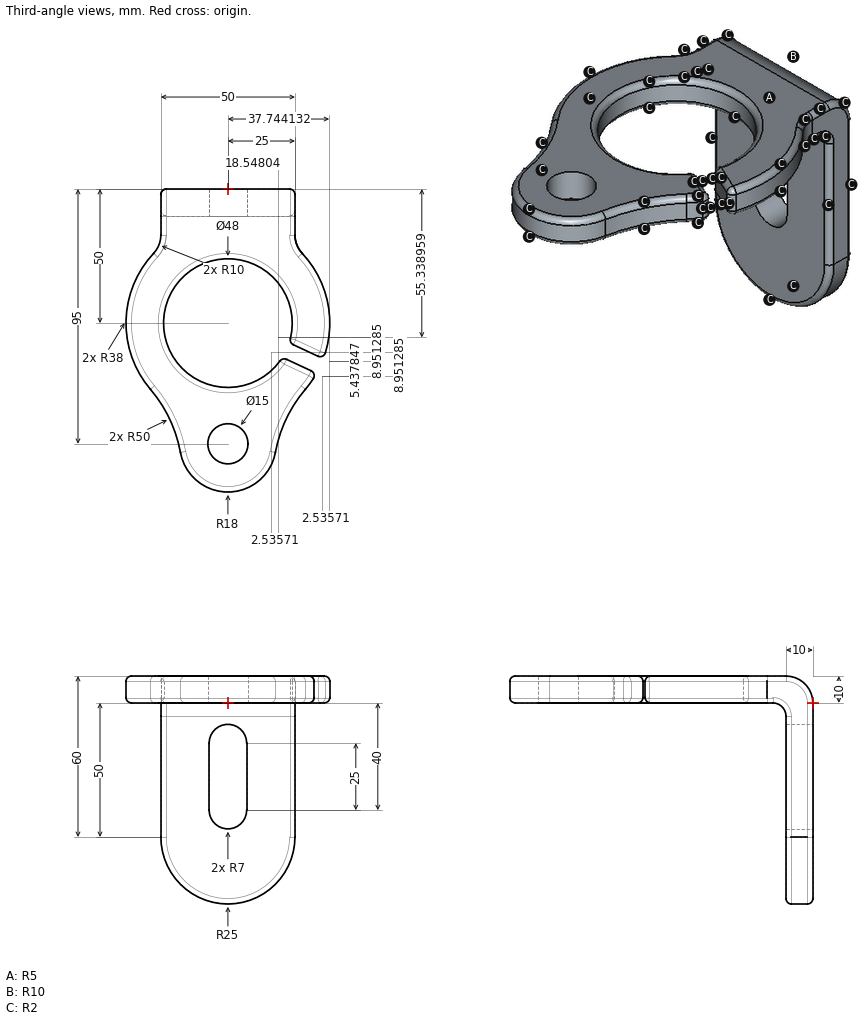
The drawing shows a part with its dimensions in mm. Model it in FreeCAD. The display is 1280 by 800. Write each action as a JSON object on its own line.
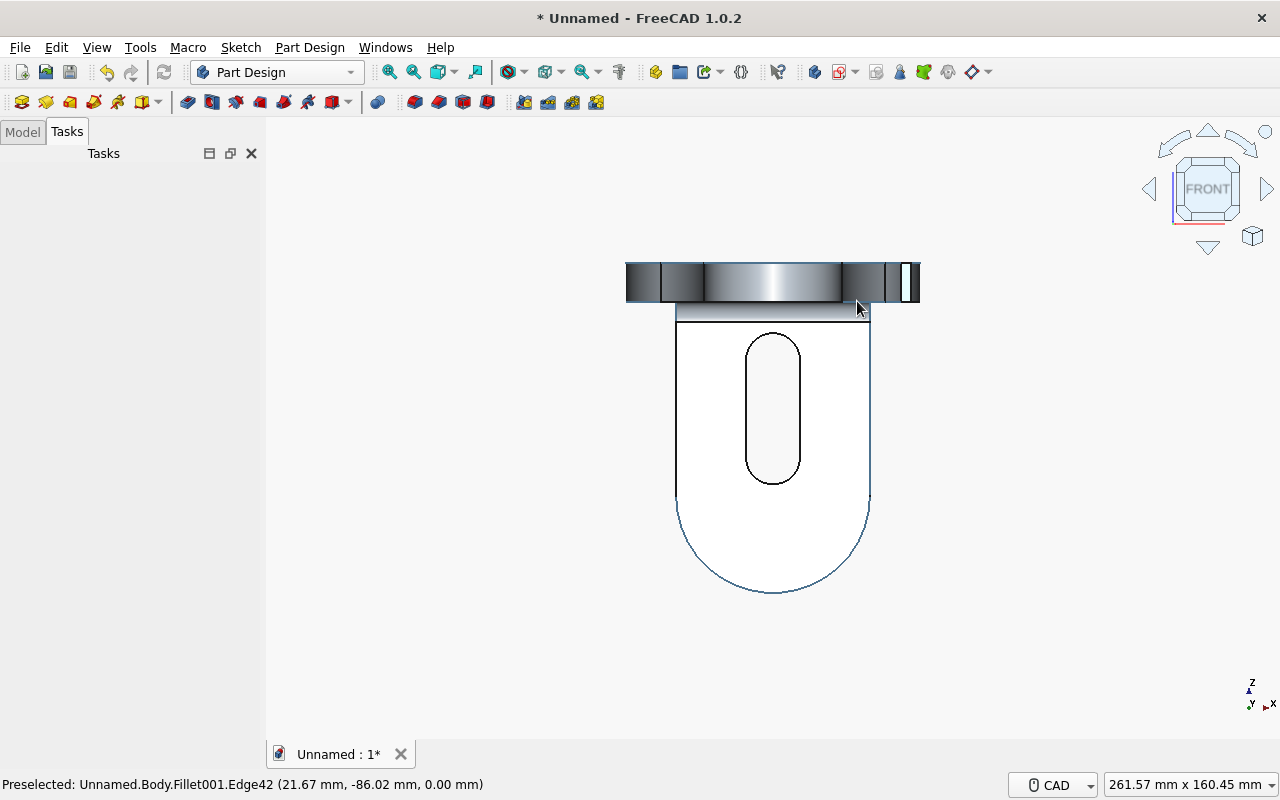
{"action": "left_click", "coordinate": [773, 301], "text": "ctrl"}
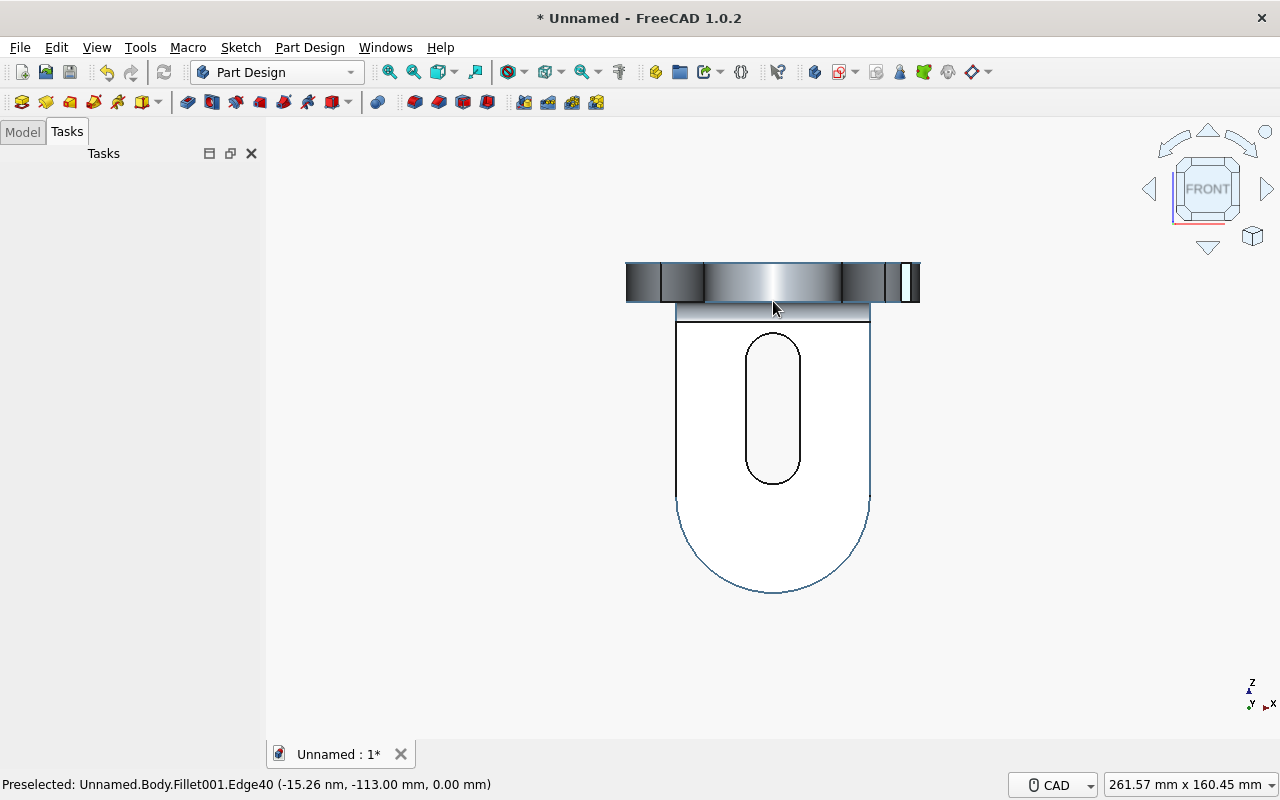
{"action": "left_click", "coordinate": [689, 301], "text": "ctrl"}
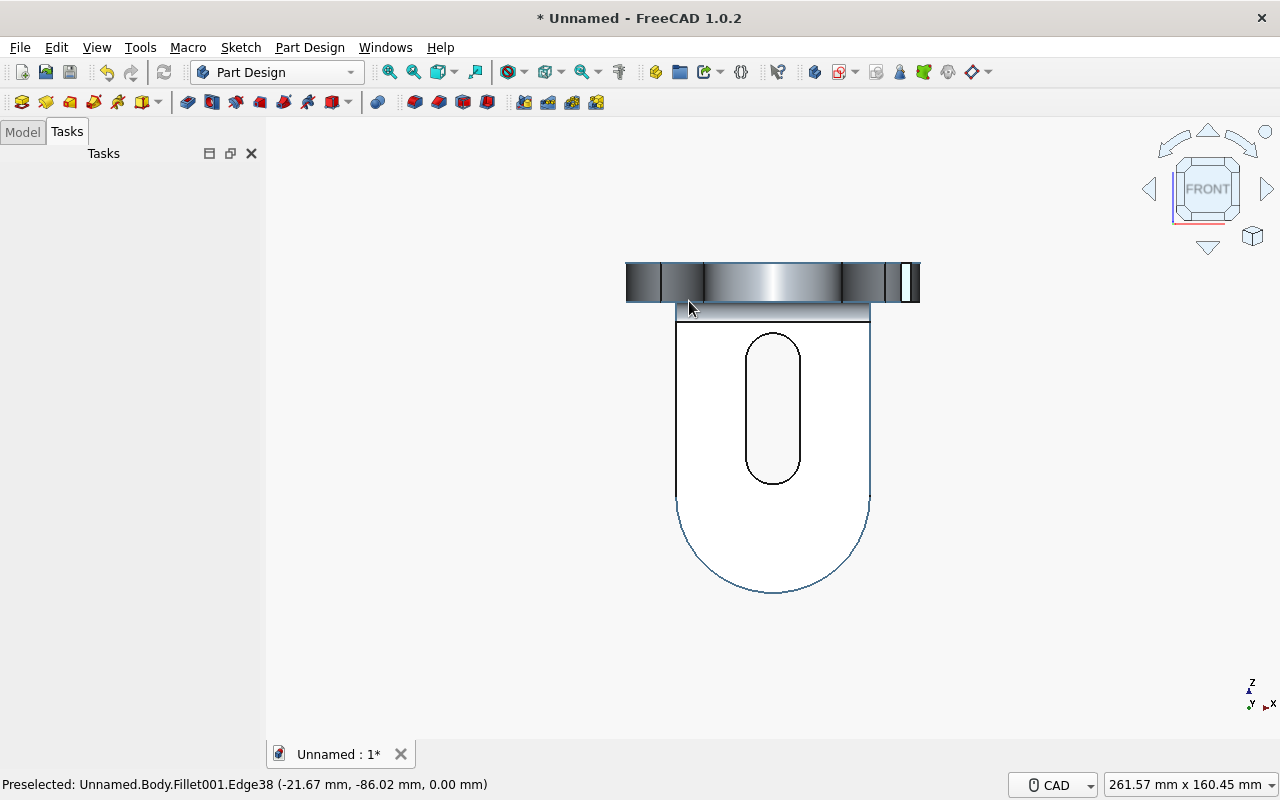
{"action": "left_click", "coordinate": [676, 408], "text": "ctrl"}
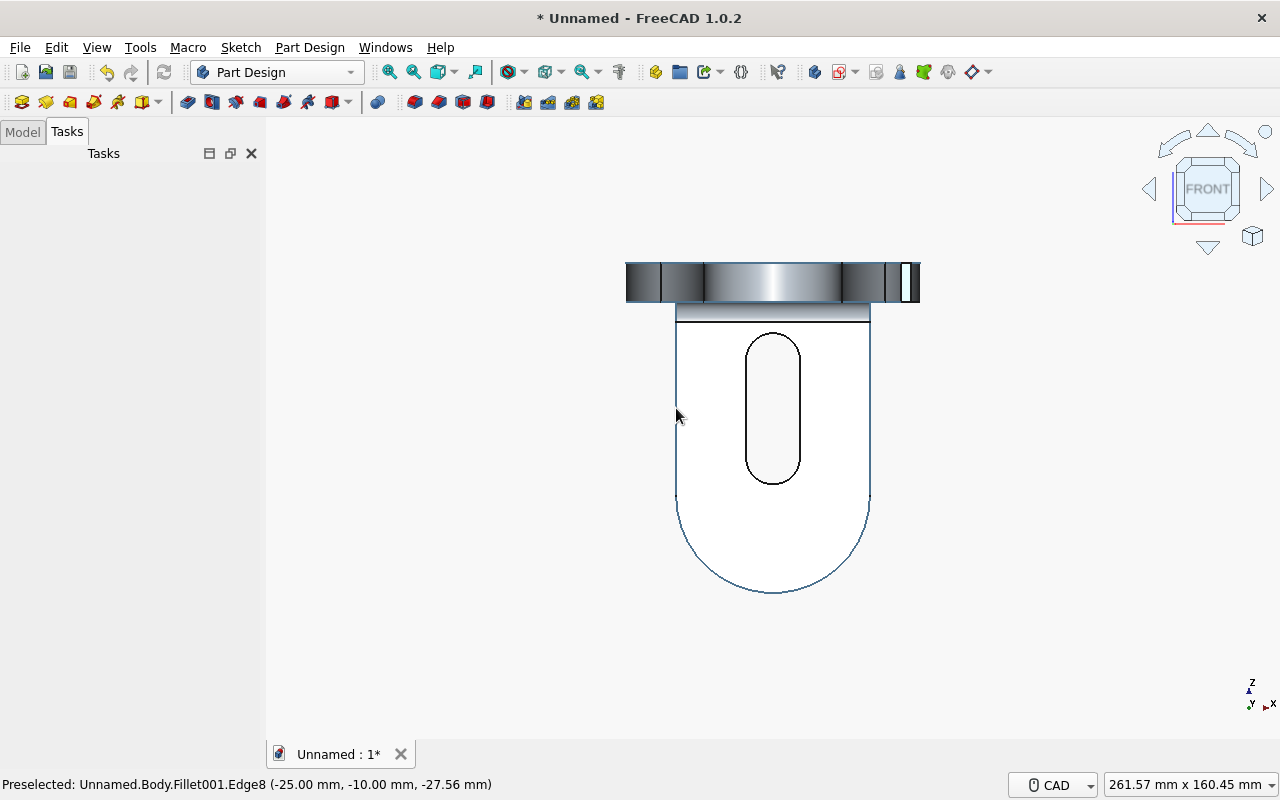
{"action": "left_click", "coordinate": [919, 301], "text": "ctrl"}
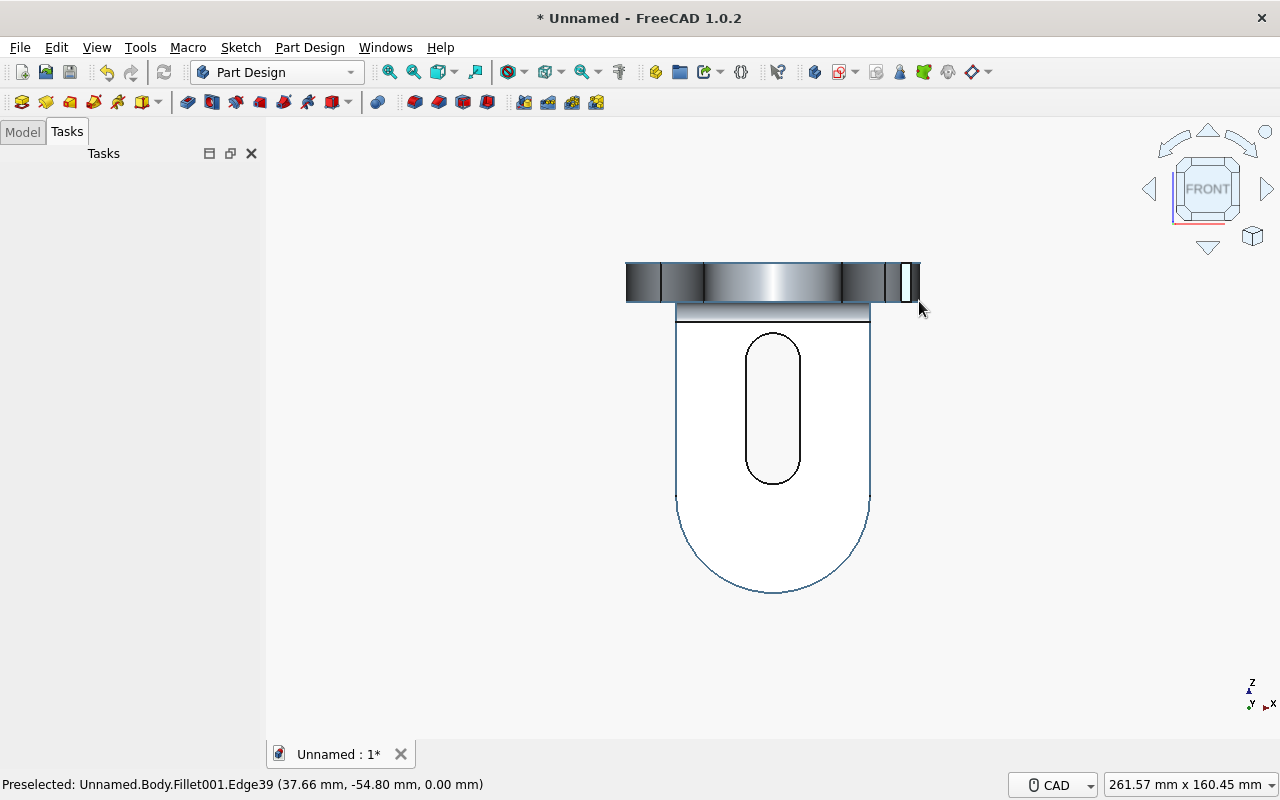
{"action": "key", "text": "3"}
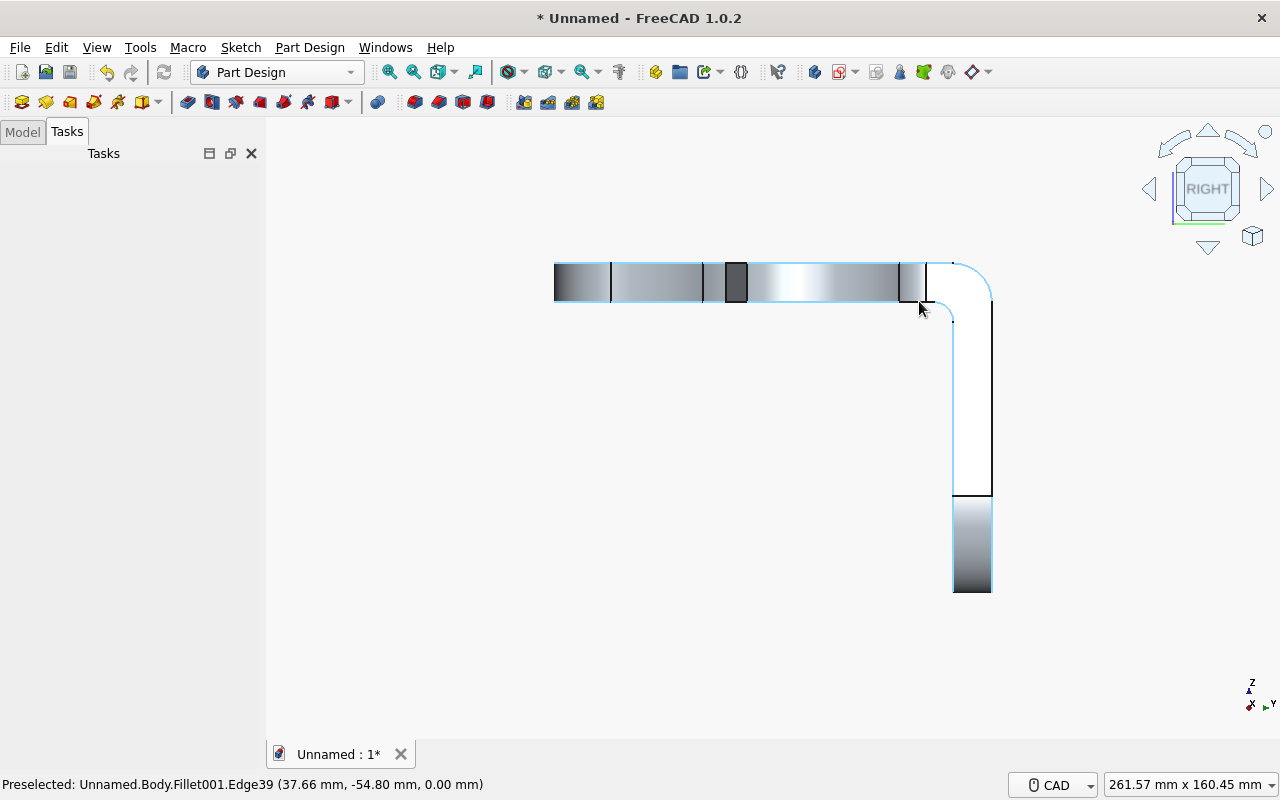
{"action": "left_click", "coordinate": [734, 282], "text": "ctrl"}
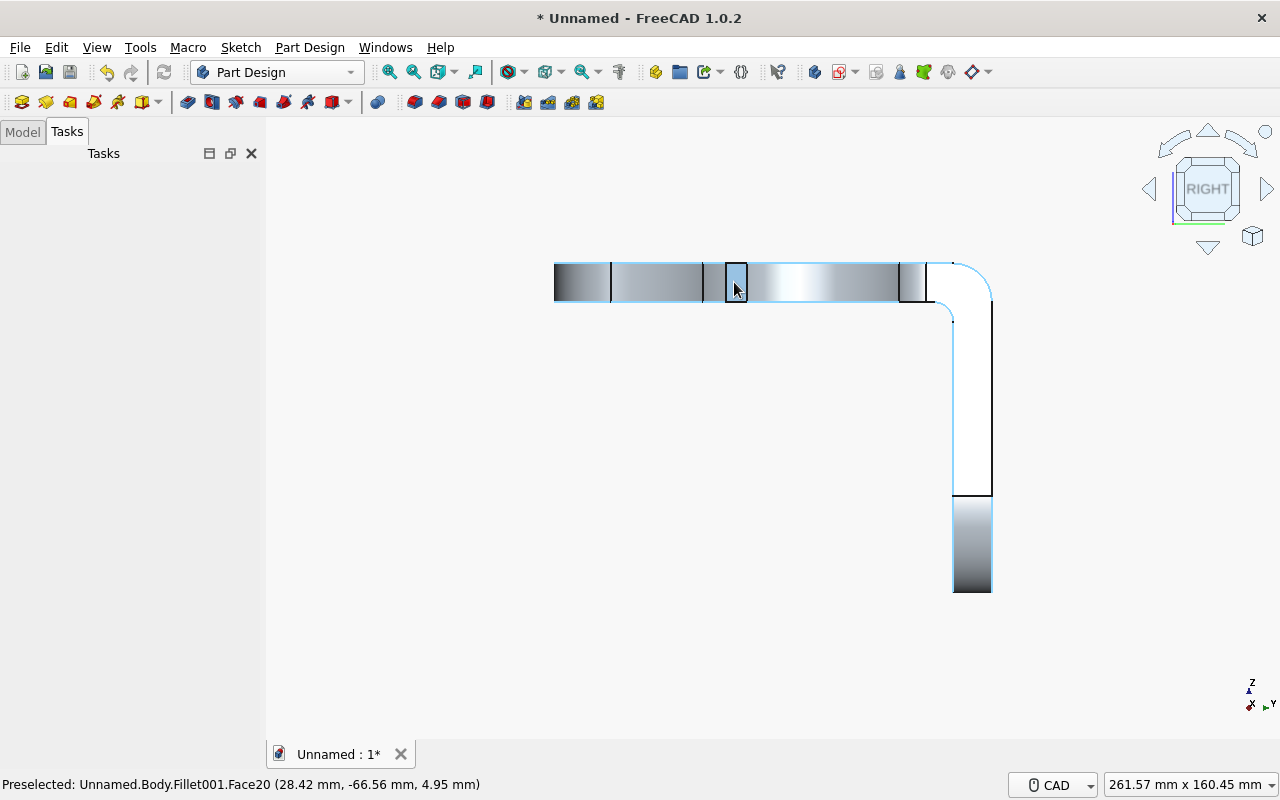
{"action": "left_click", "coordinate": [992, 398], "text": "ctrl"}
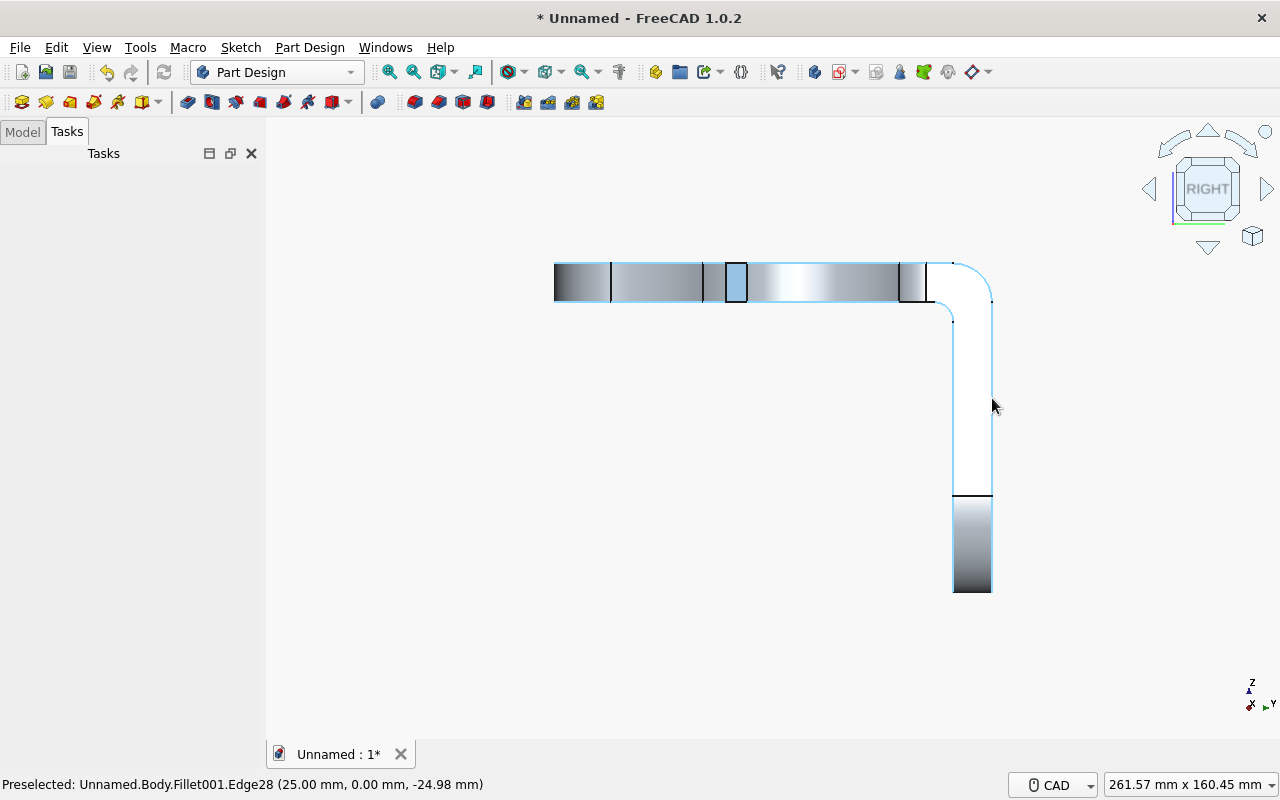
{"action": "left_click", "coordinate": [911, 301], "text": "ctrl"}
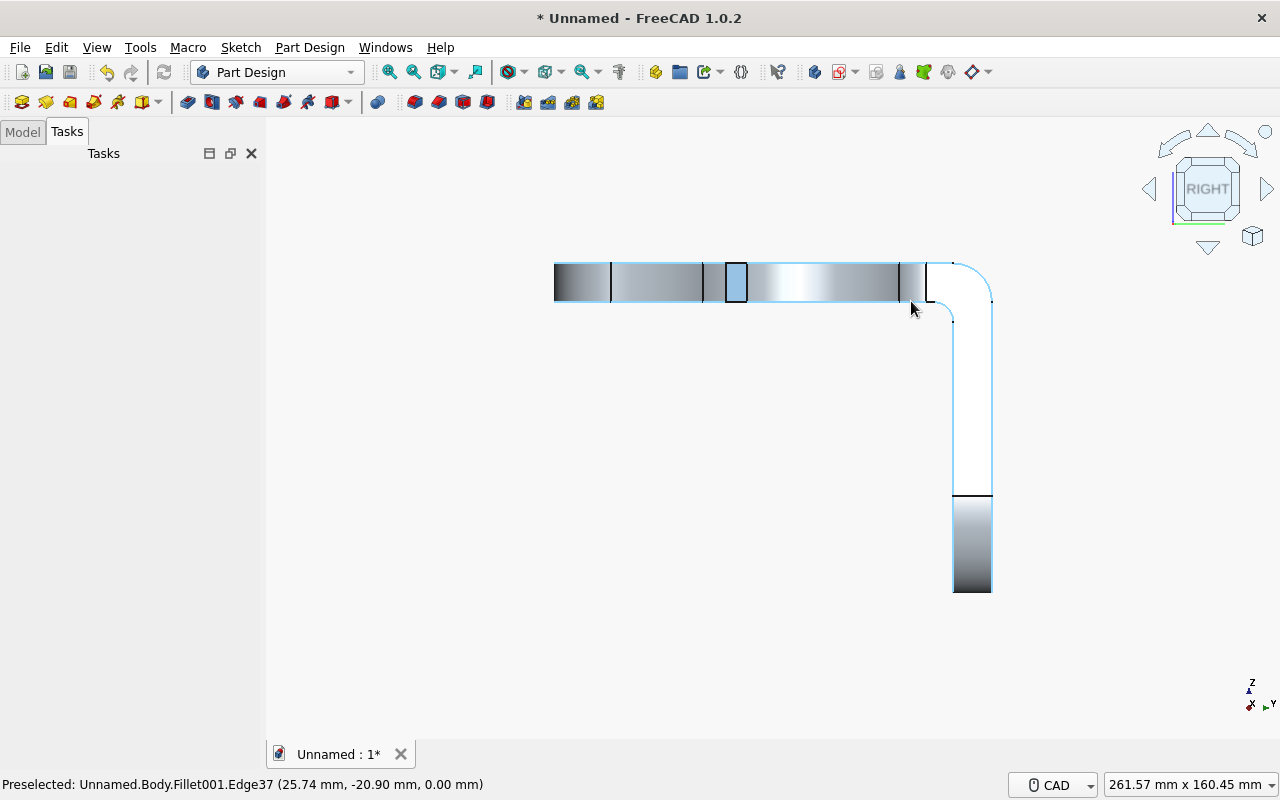
{"action": "scroll", "coordinate": [930, 301], "scroll_direction": "up", "scroll_amount": 8}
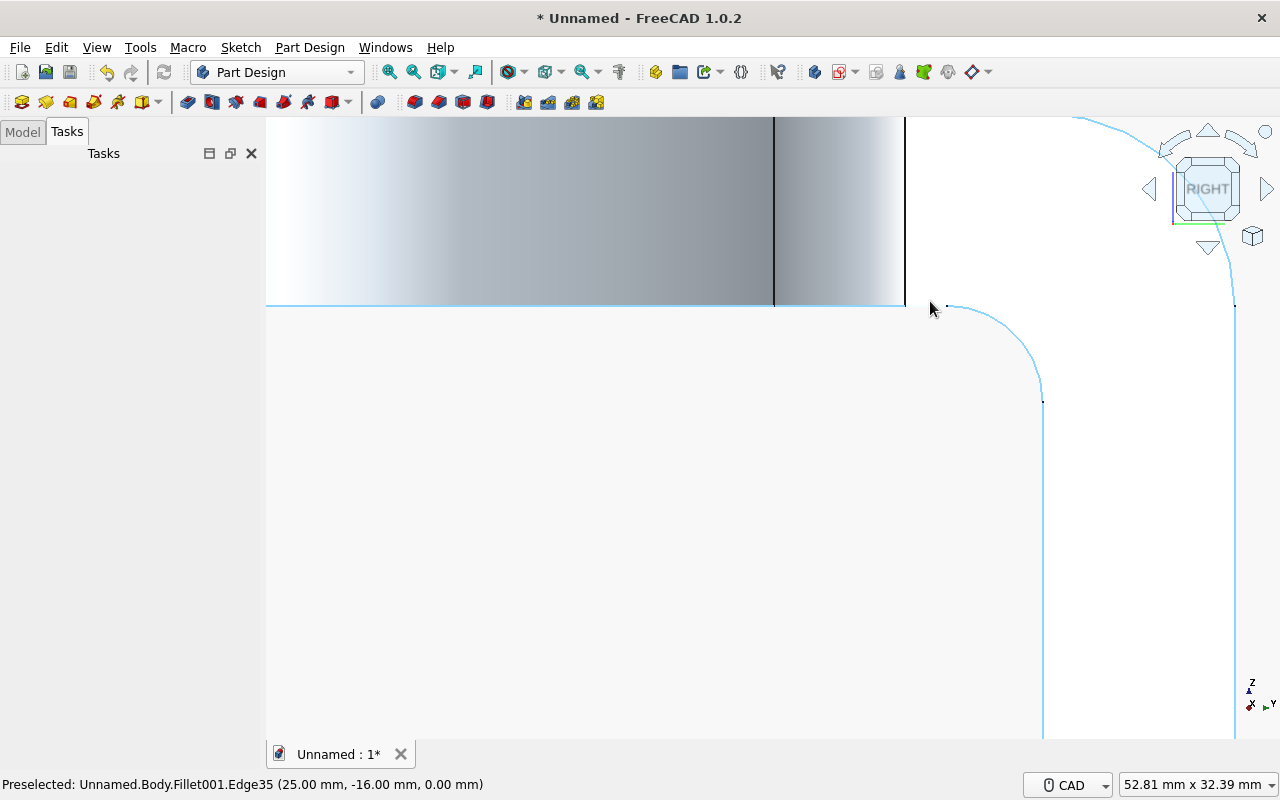
{"action": "left_click", "coordinate": [926, 305], "text": "ctrl"}